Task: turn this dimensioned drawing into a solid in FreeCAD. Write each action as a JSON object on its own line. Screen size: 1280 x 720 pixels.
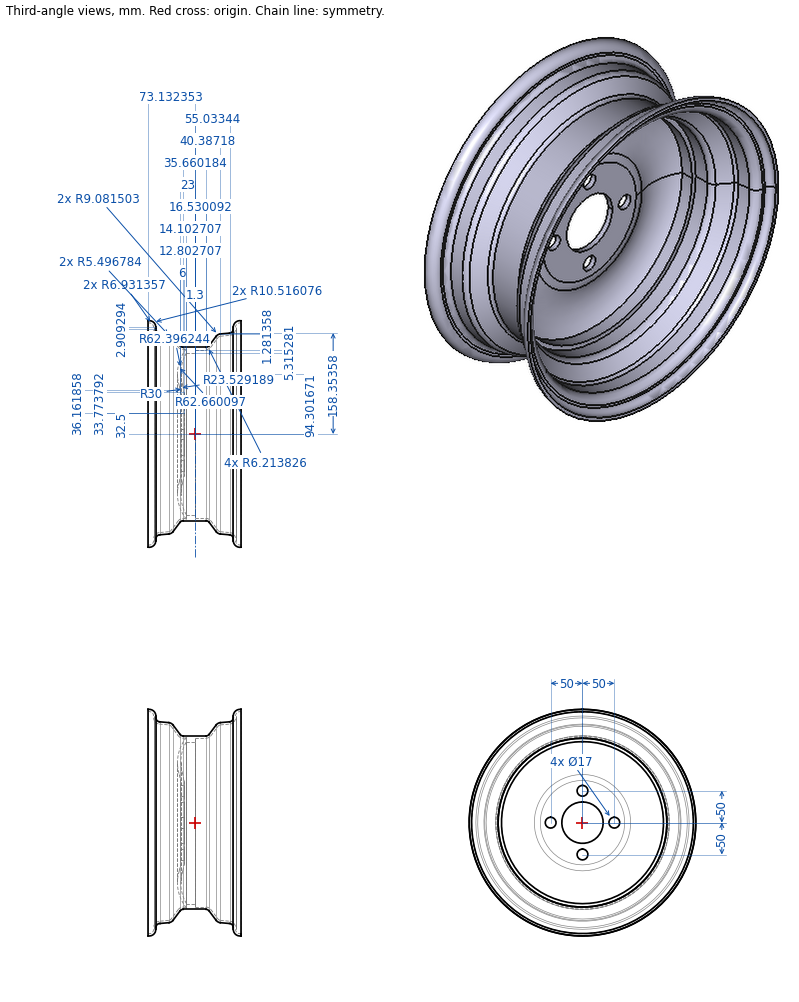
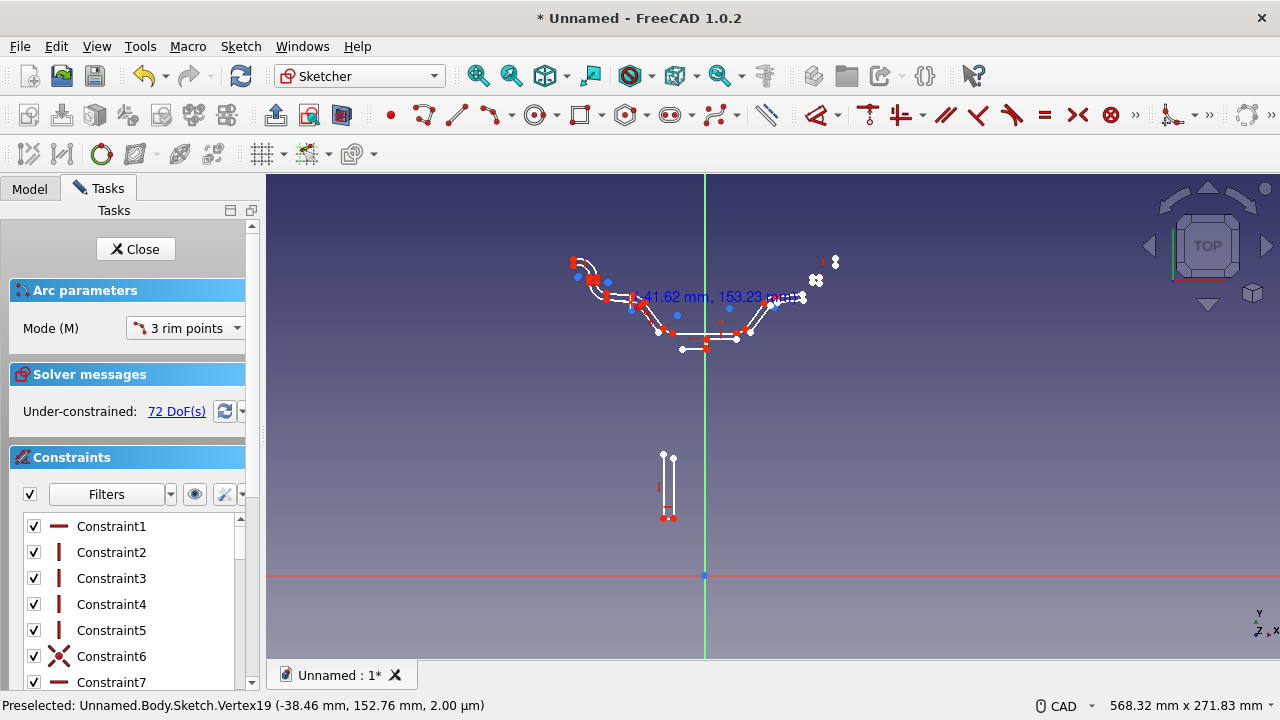
{"action": "scroll", "coordinate": [659, 332], "scroll_direction": "up", "scroll_amount": 5}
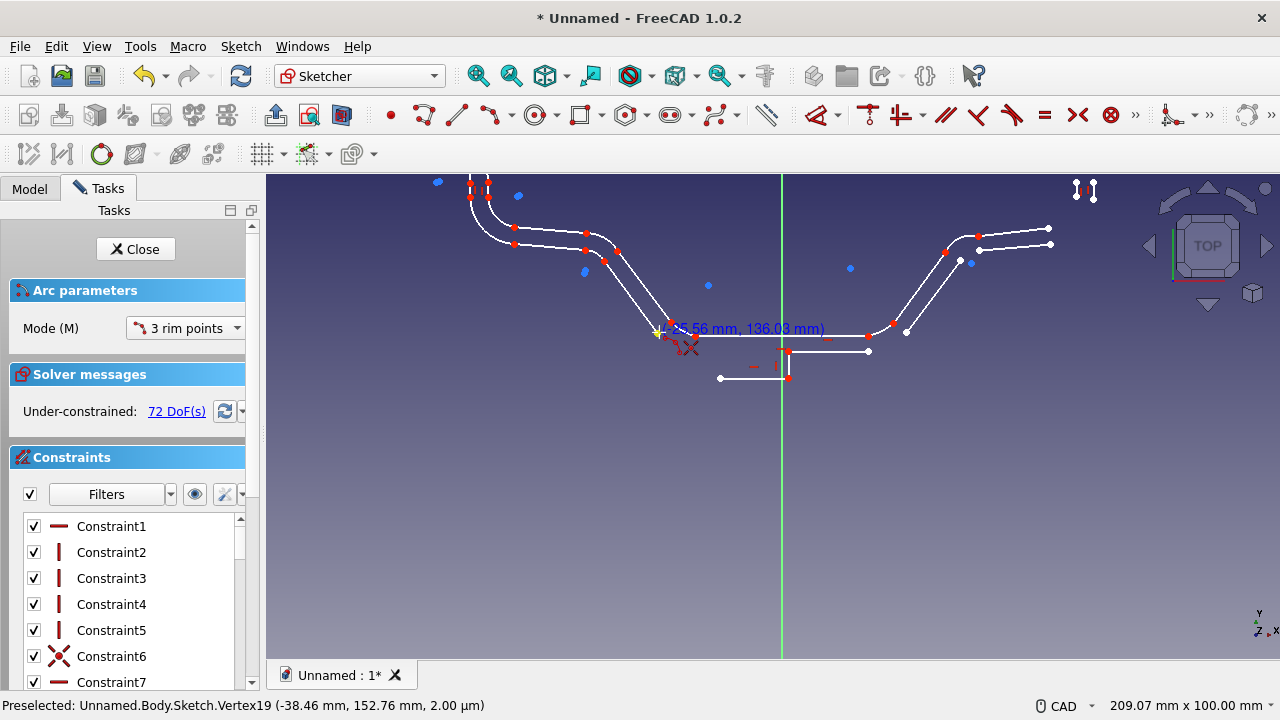
{"action": "left_click", "coordinate": [657, 333]}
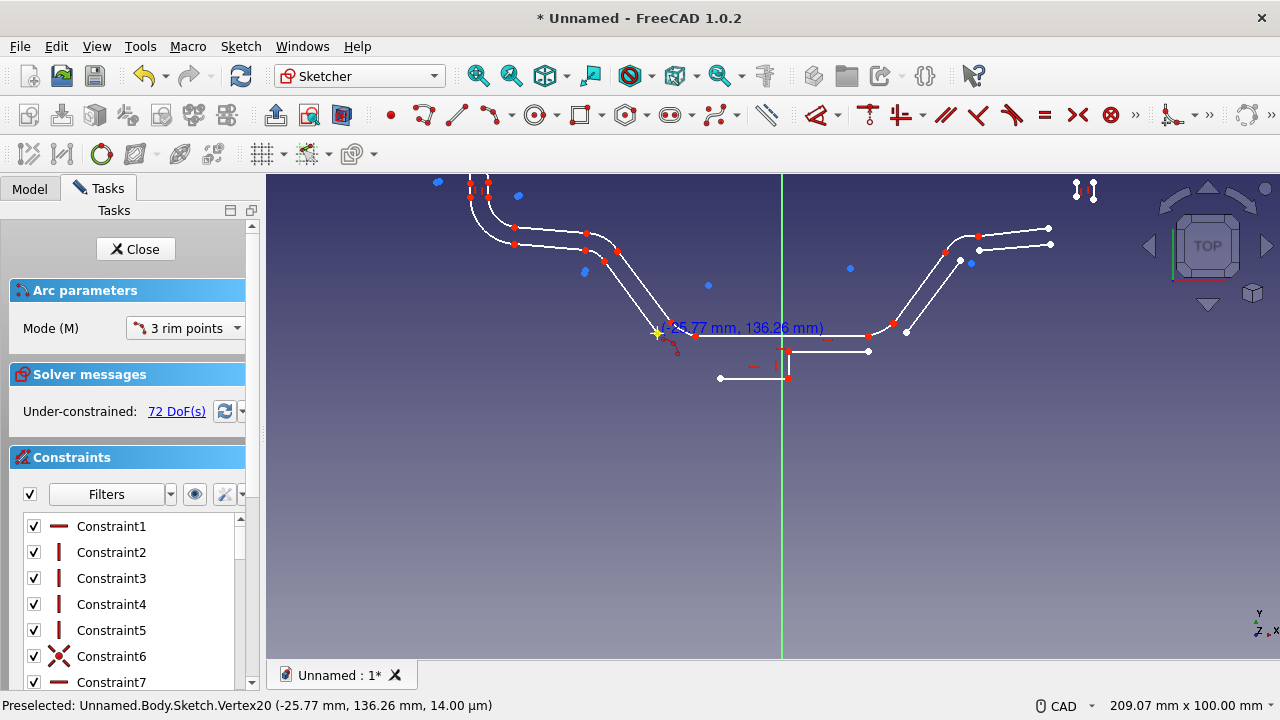
{"action": "scroll", "coordinate": [720, 344], "scroll_direction": "up", "scroll_amount": 2}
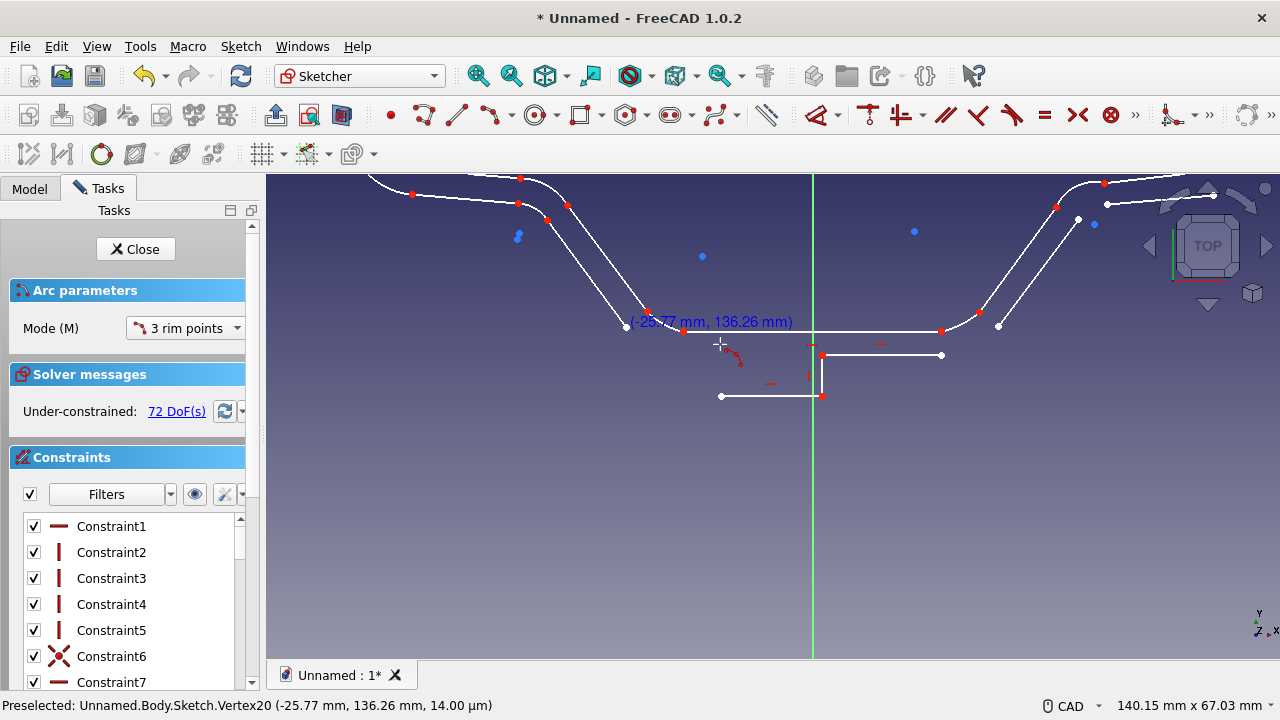
{"action": "left_click", "coordinate": [720, 345]}
{"action": "left_click", "coordinate": [670, 353]}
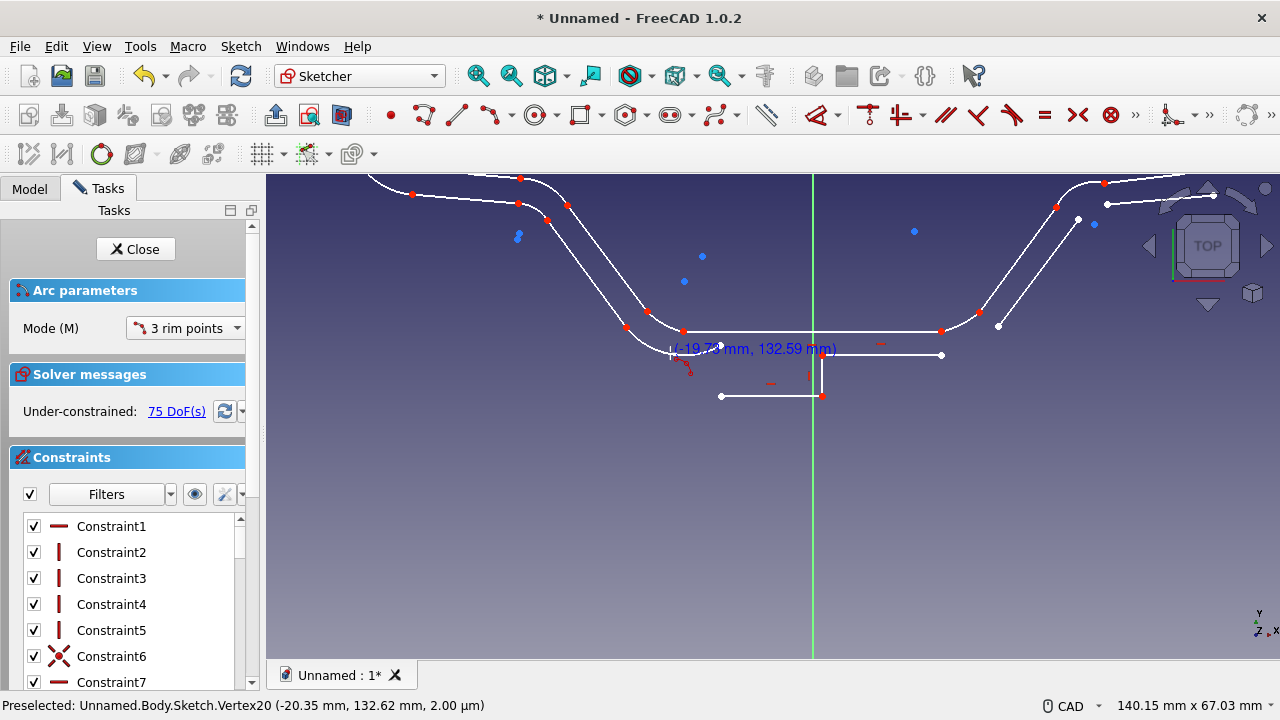
{"action": "left_click", "coordinate": [720, 346]}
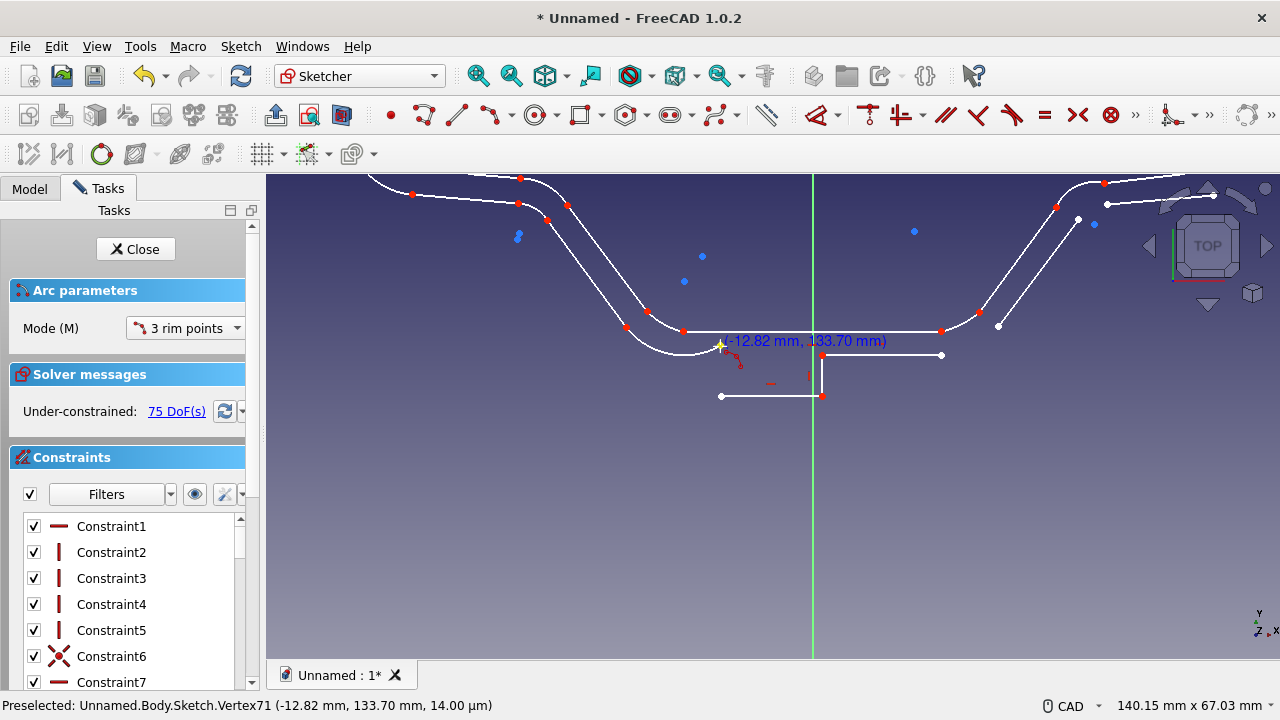
{"action": "scroll", "coordinate": [669, 333], "scroll_direction": "down", "scroll_amount": 7}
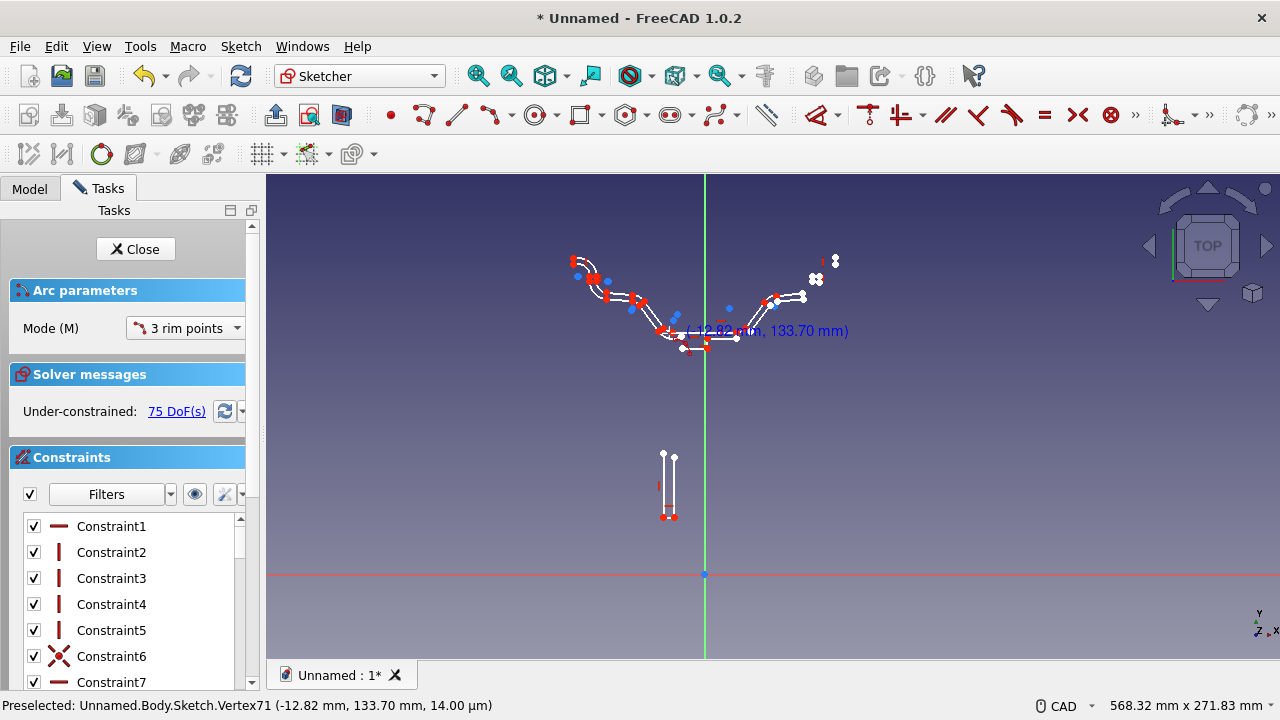
{"action": "scroll", "coordinate": [662, 440], "scroll_direction": "up", "scroll_amount": 2}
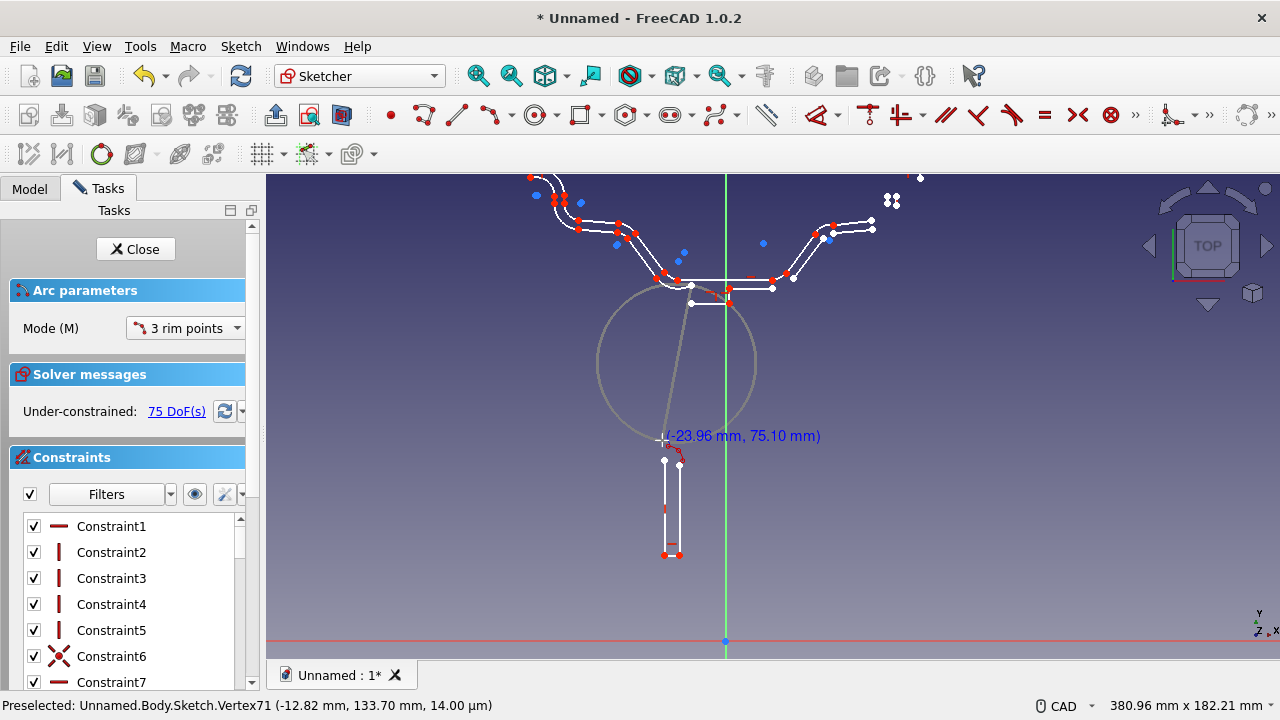
{"action": "left_click", "coordinate": [662, 440]}
{"action": "left_click", "coordinate": [657, 358]}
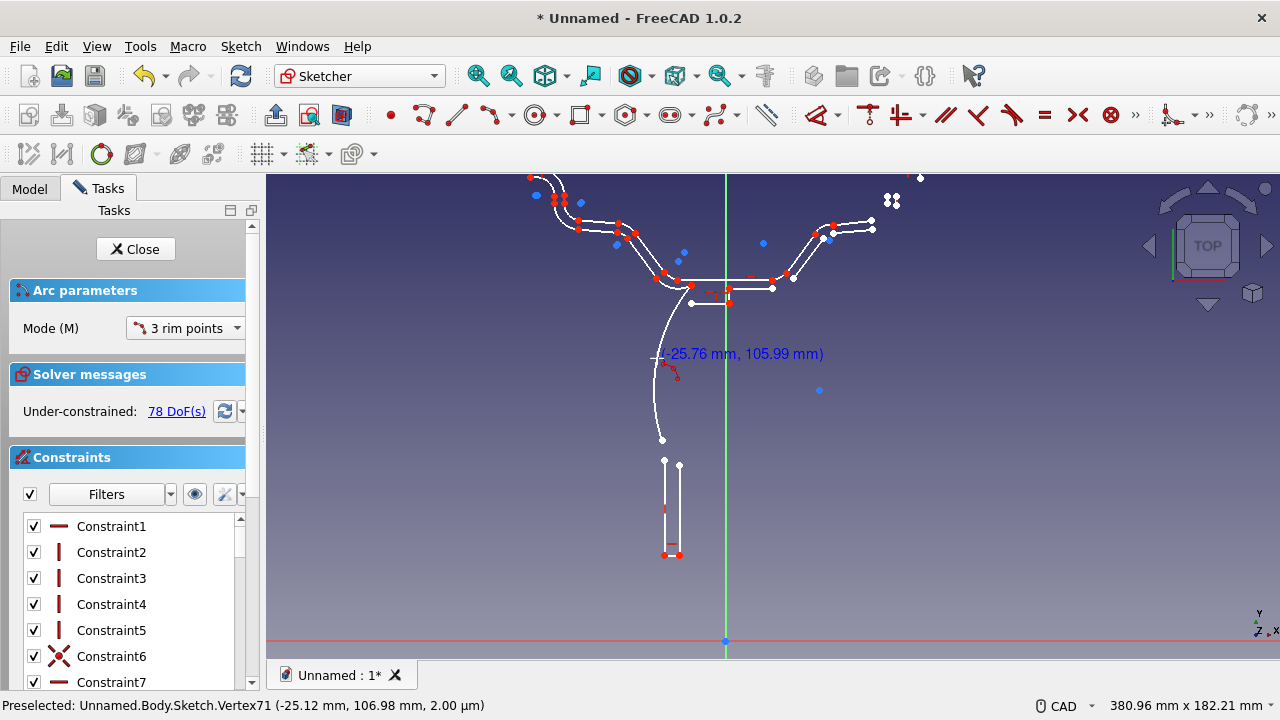
{"action": "left_click", "coordinate": [662, 441]}
{"action": "left_click", "coordinate": [665, 460]}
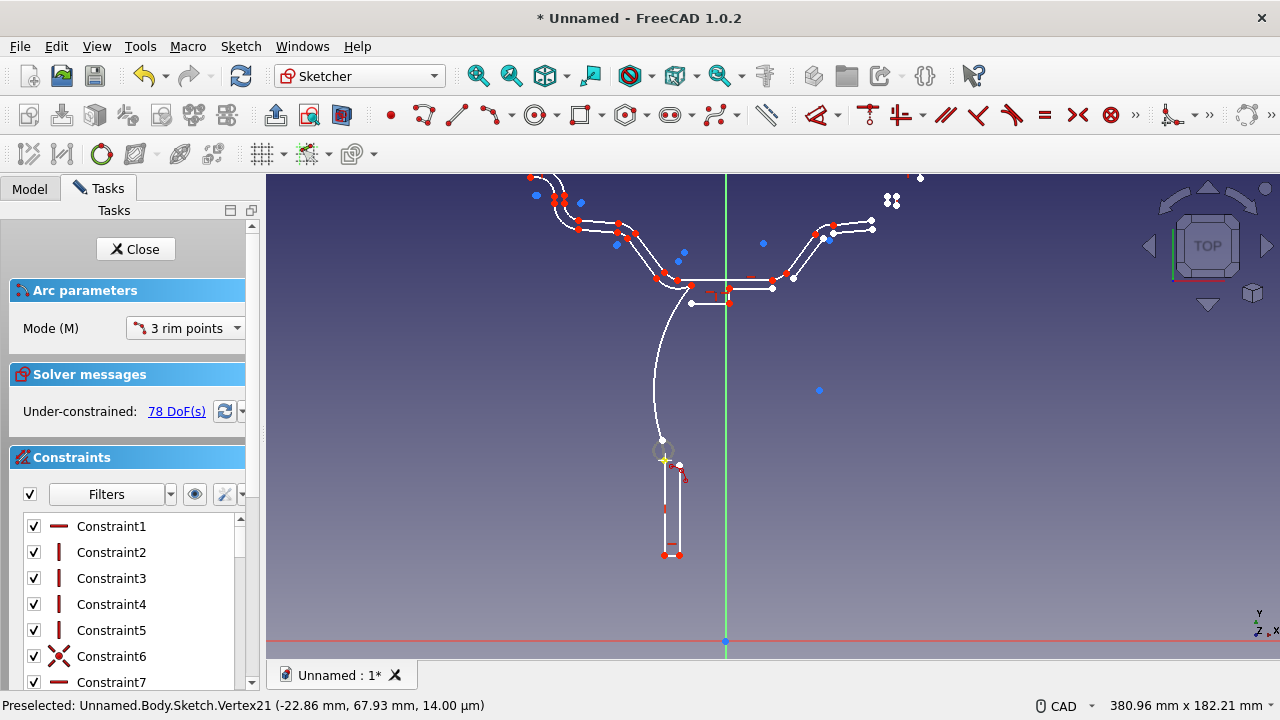
{"action": "scroll", "coordinate": [664, 449], "scroll_direction": "up", "scroll_amount": 16}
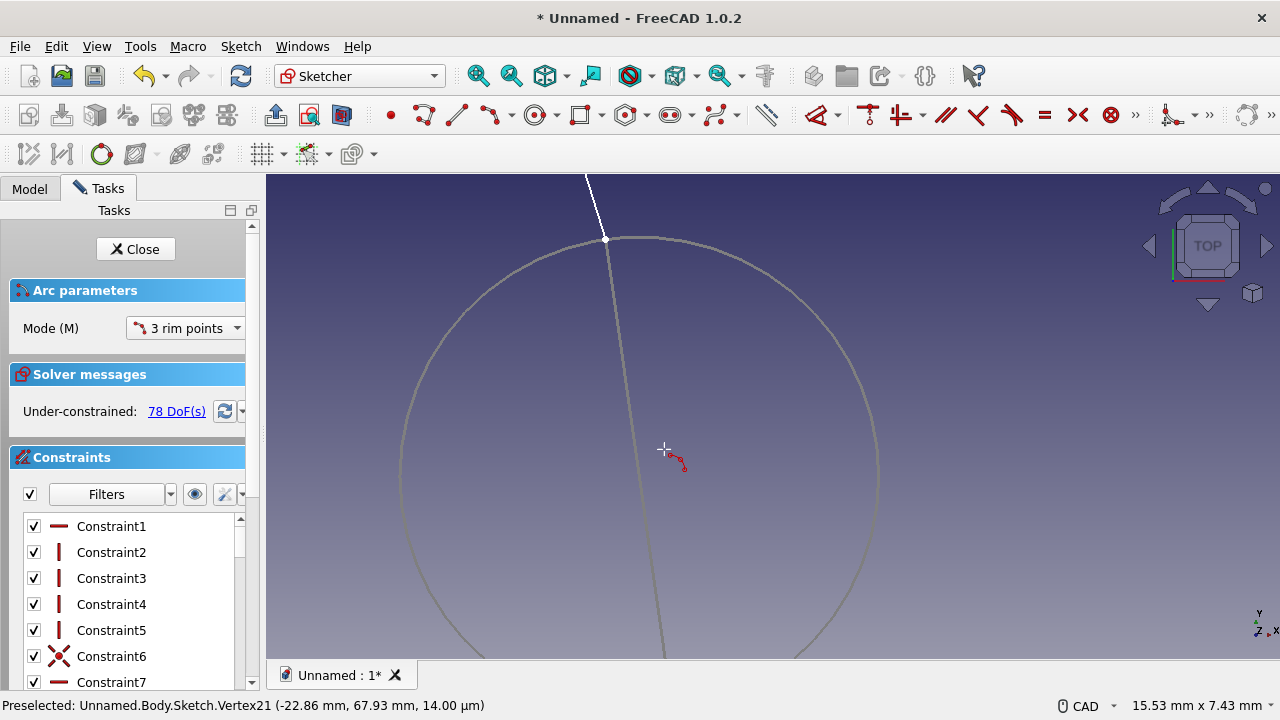
{"action": "left_click", "coordinate": [646, 434]}